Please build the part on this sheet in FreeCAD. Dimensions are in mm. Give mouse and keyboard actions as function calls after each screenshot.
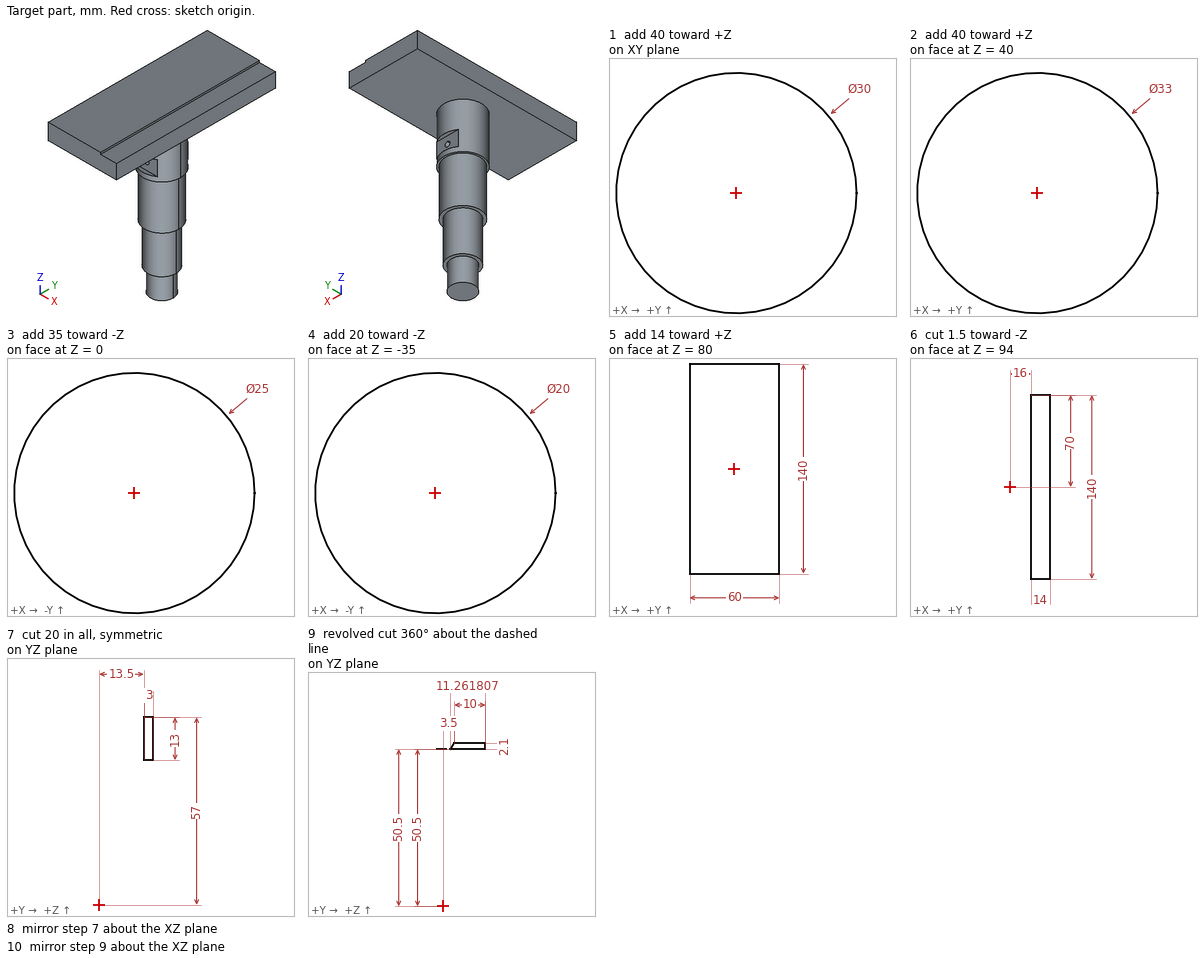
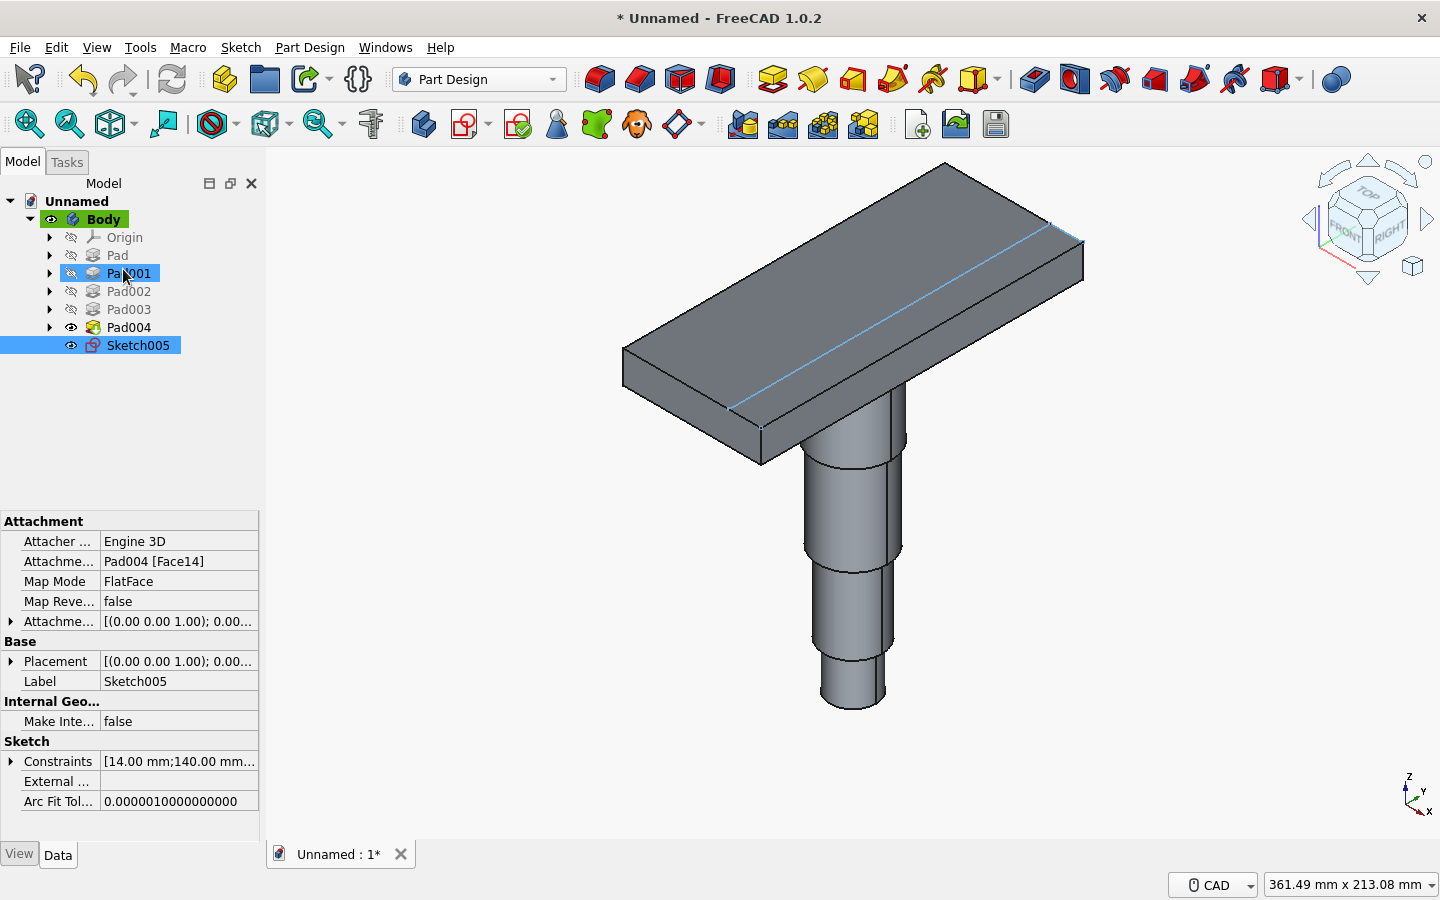
click(1036, 80)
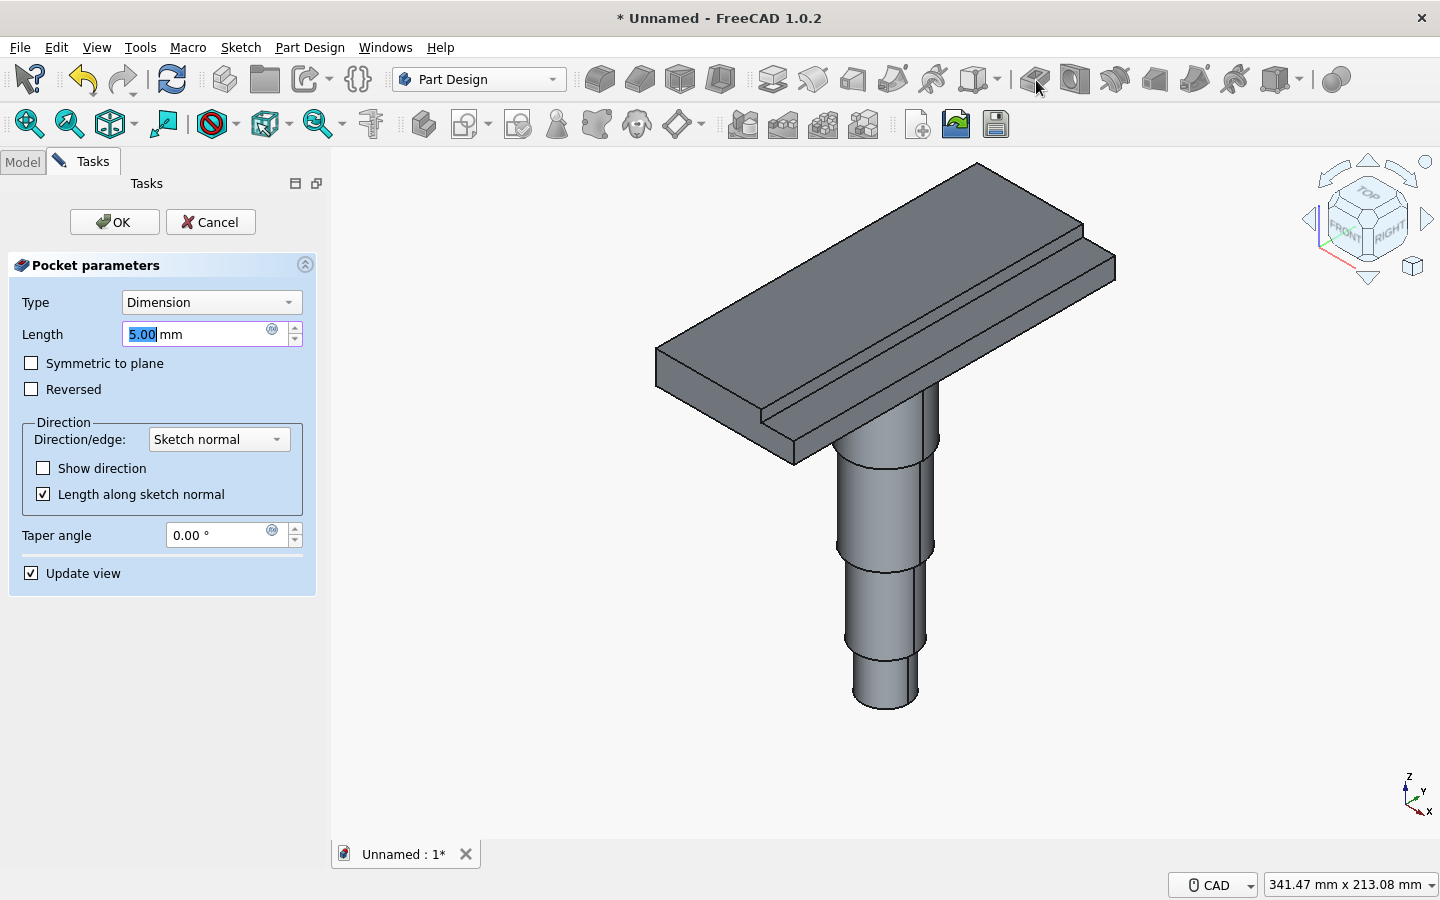
text(1.5)
key(Tab)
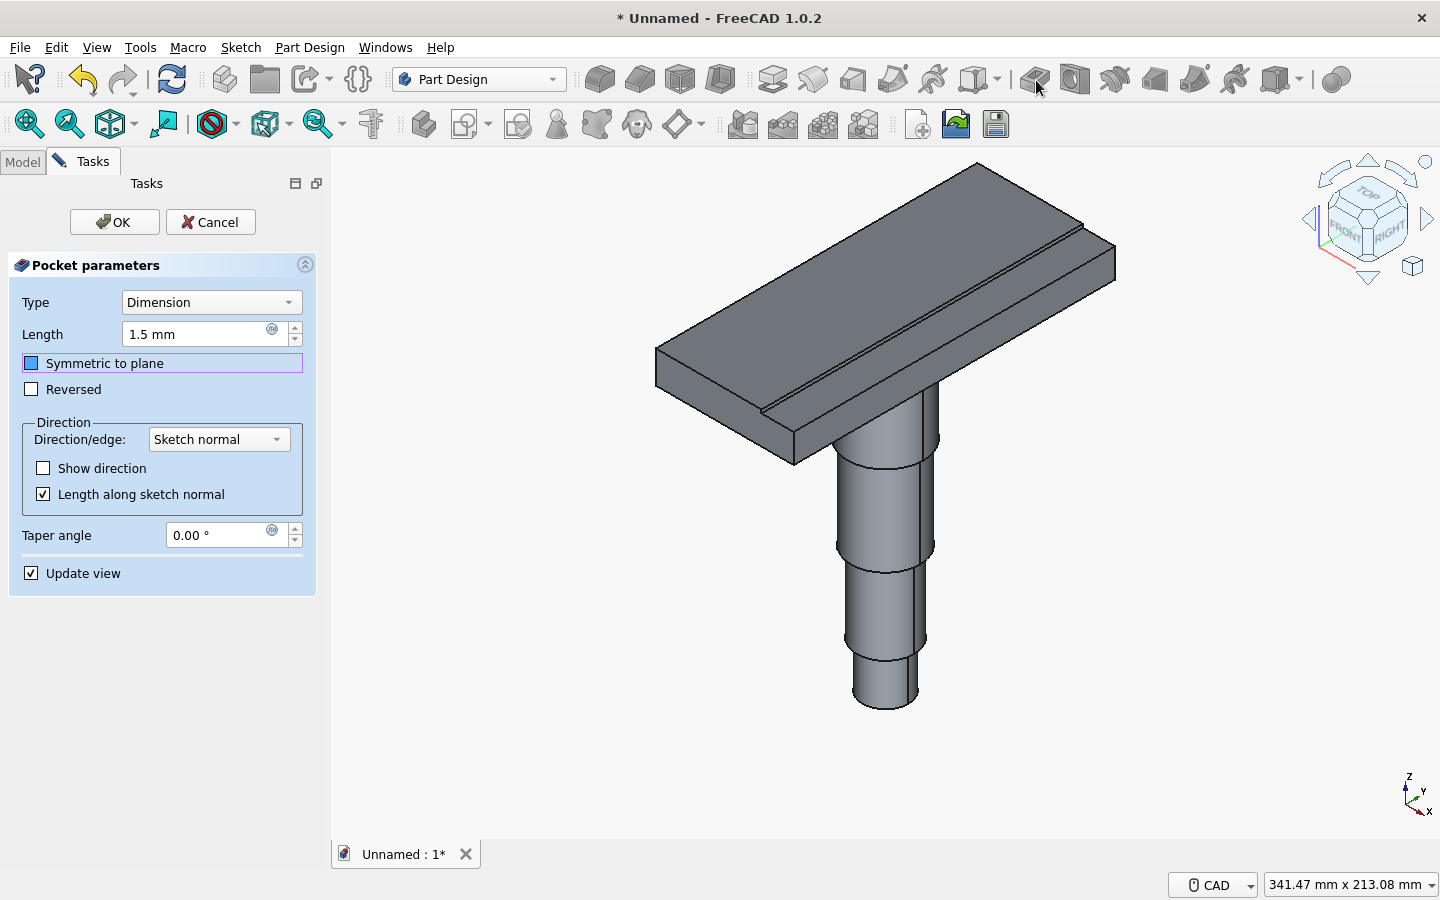
click(115, 222)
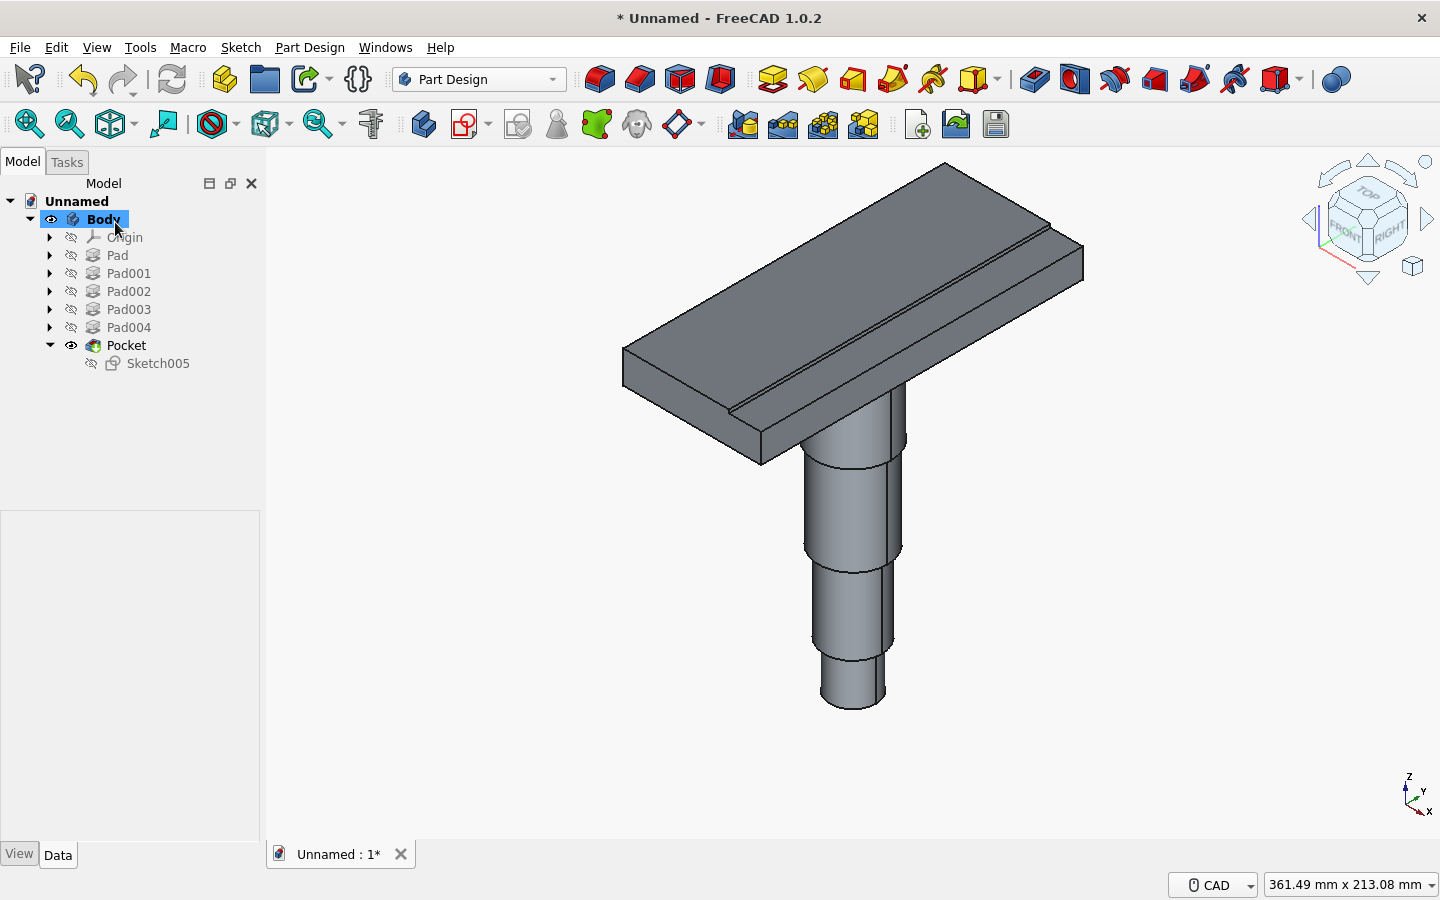
click(464, 124)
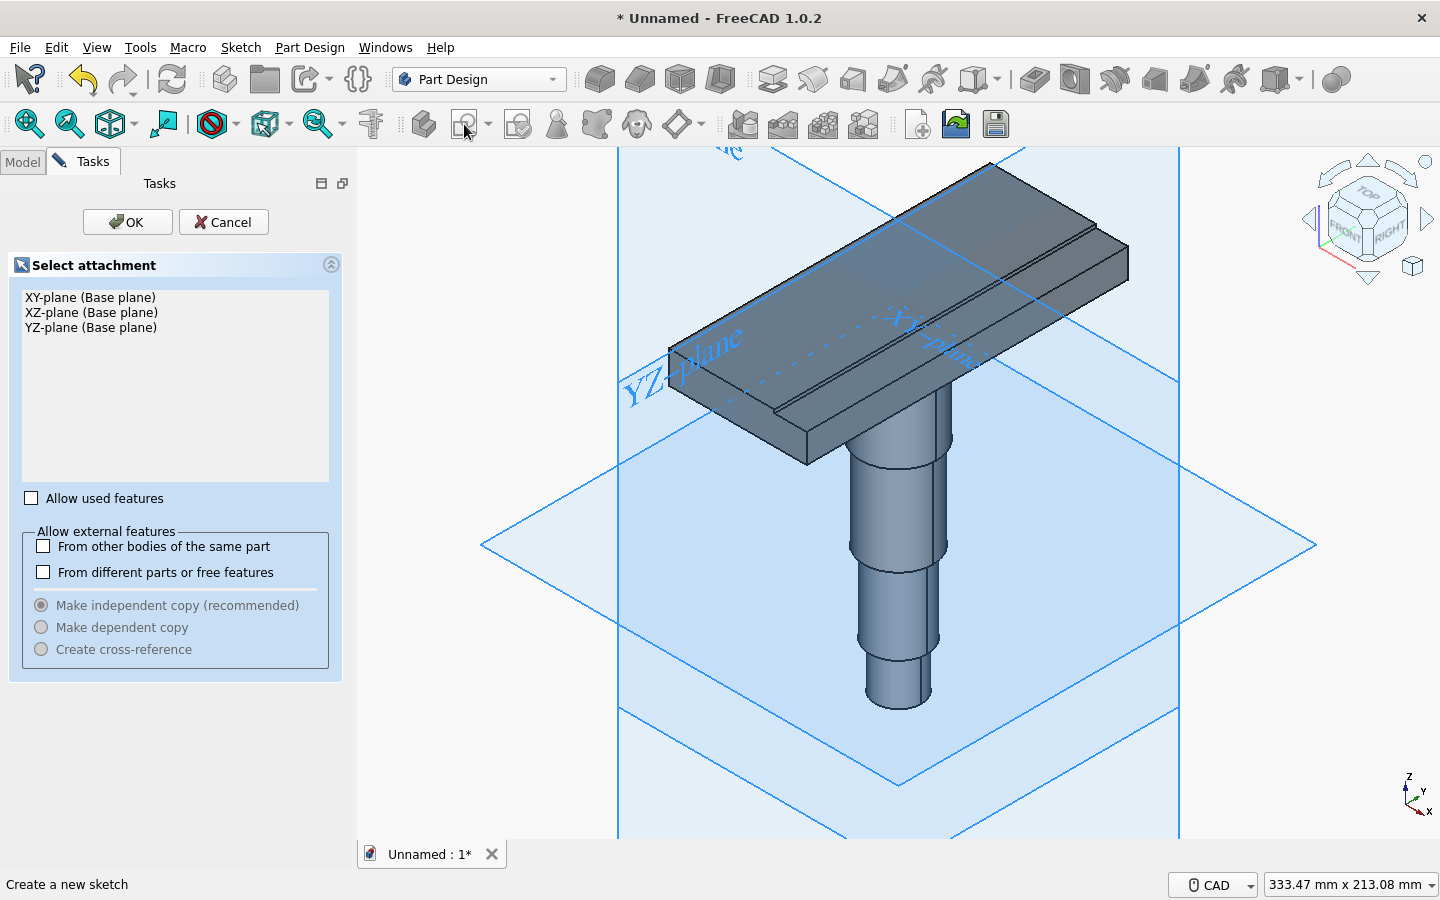
click(82, 328)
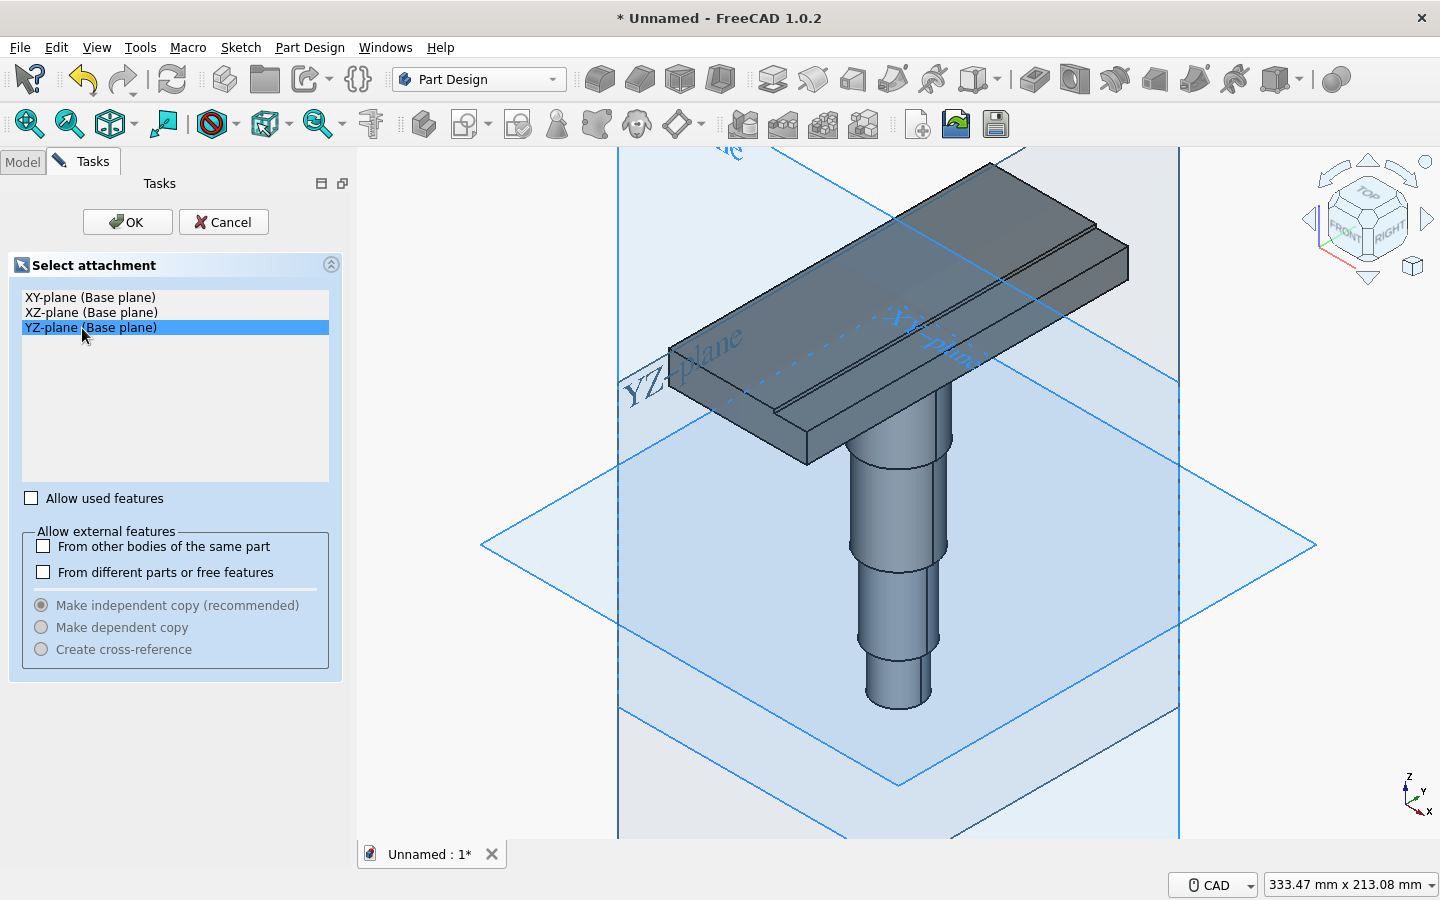
click(128, 222)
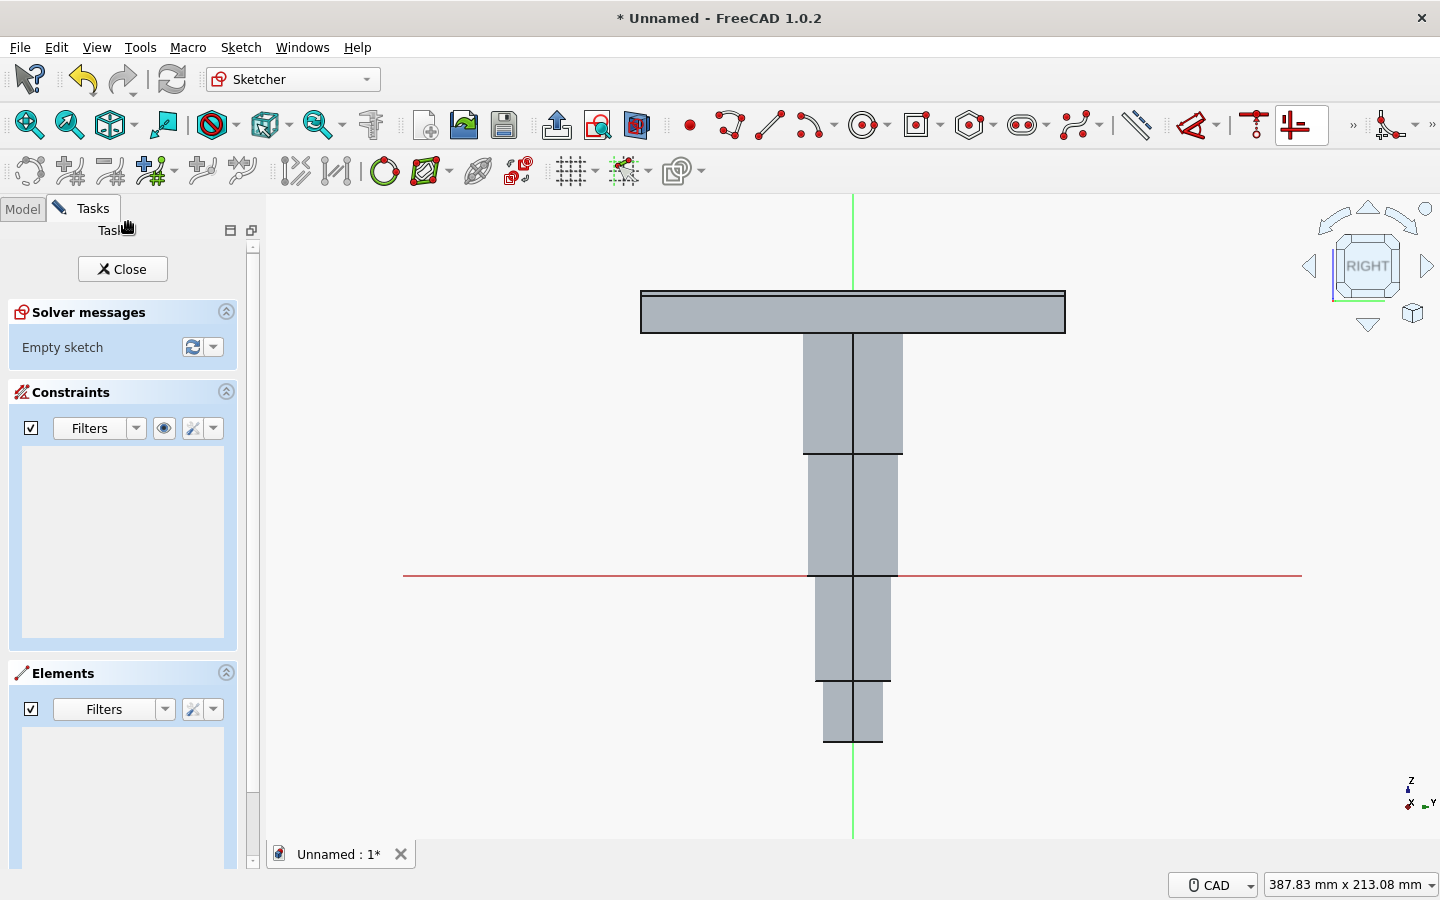
click(638, 126)